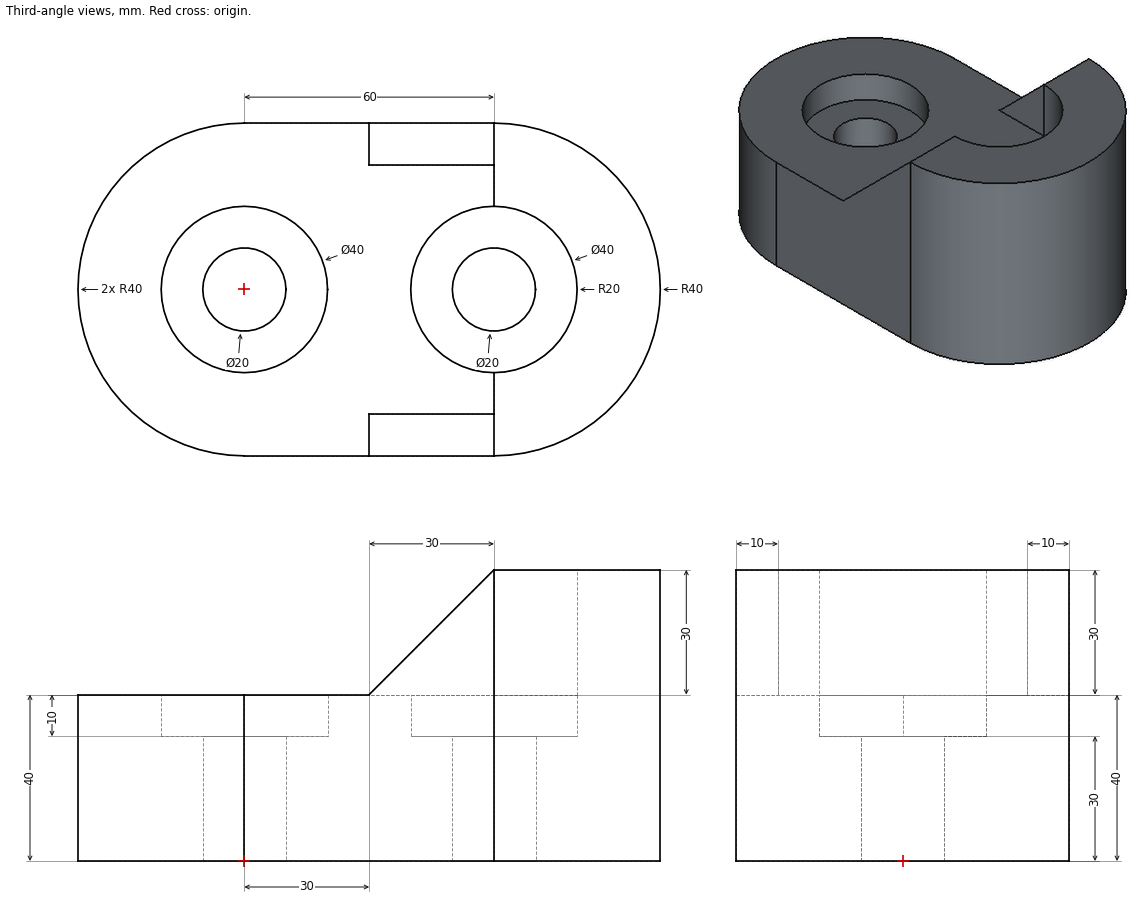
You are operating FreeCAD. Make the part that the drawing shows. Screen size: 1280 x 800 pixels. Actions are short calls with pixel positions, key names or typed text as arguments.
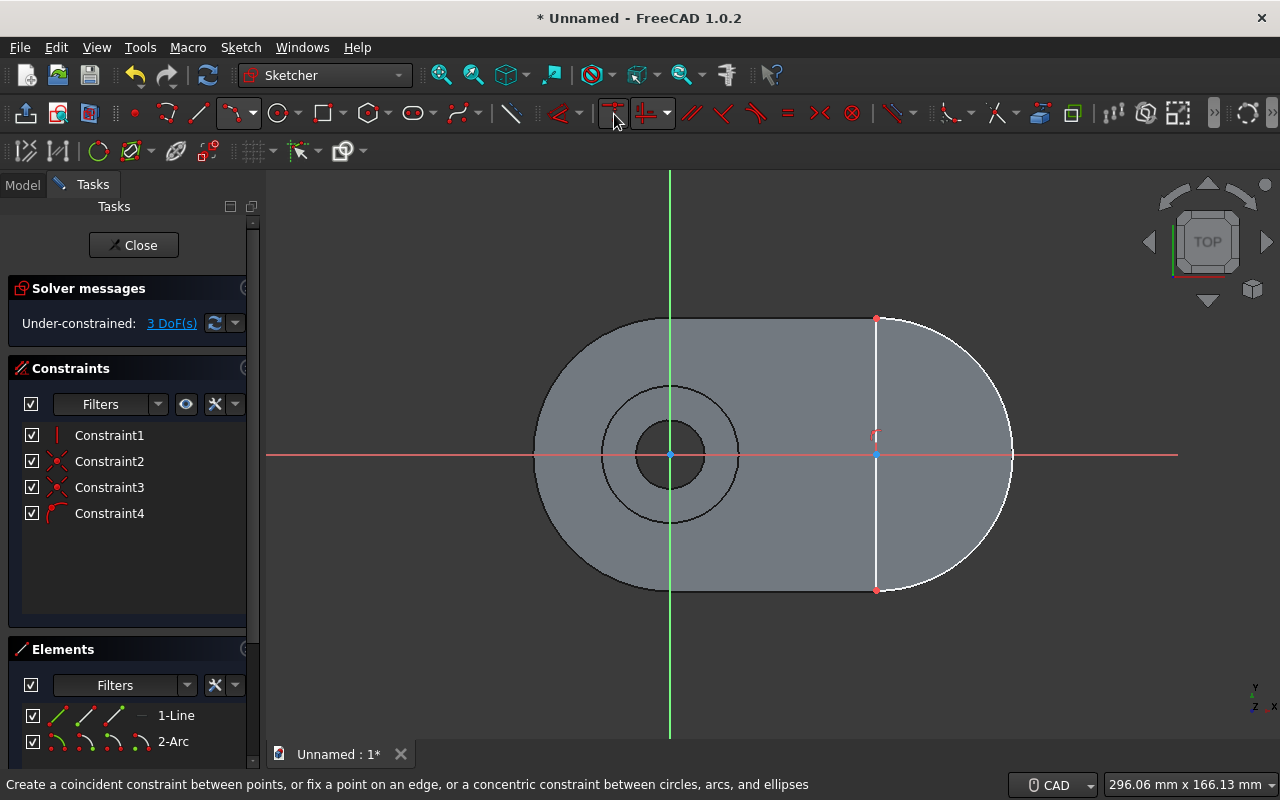
click(558, 114)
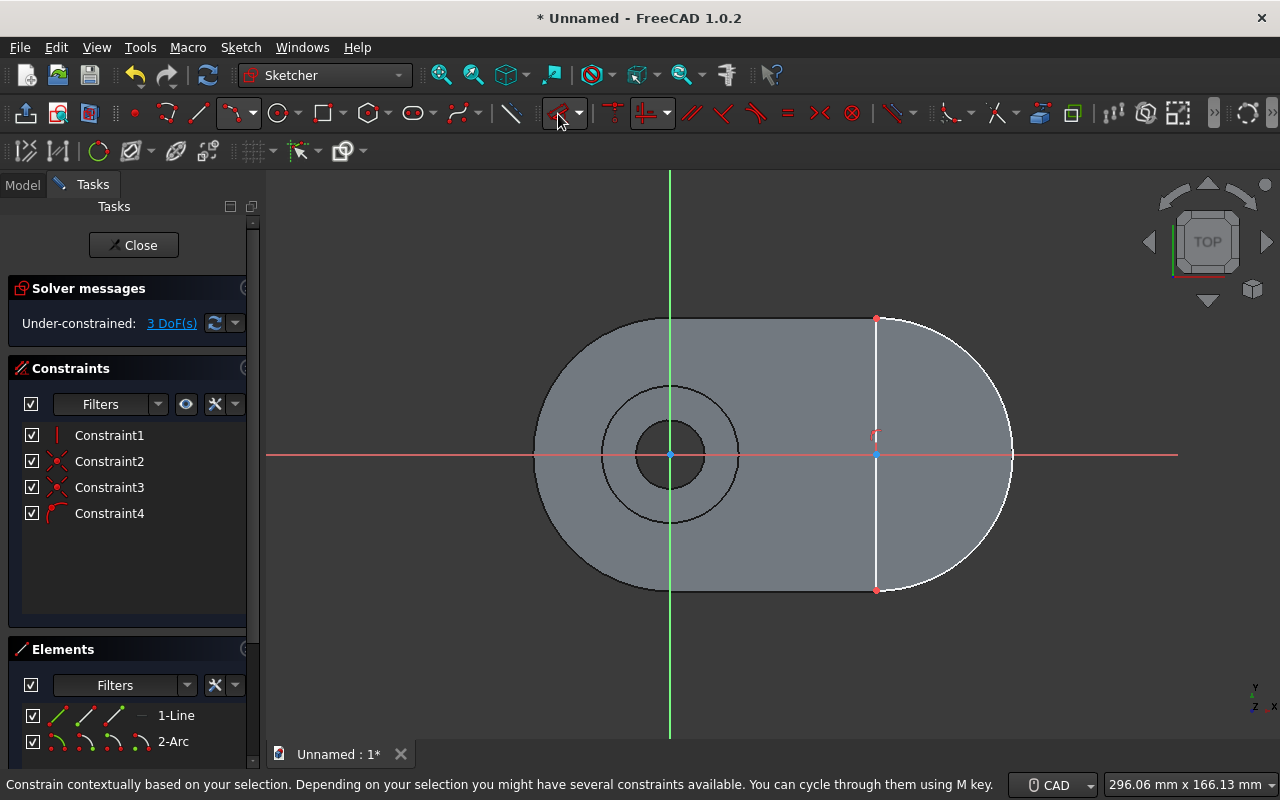
click(987, 535)
click(1013, 554)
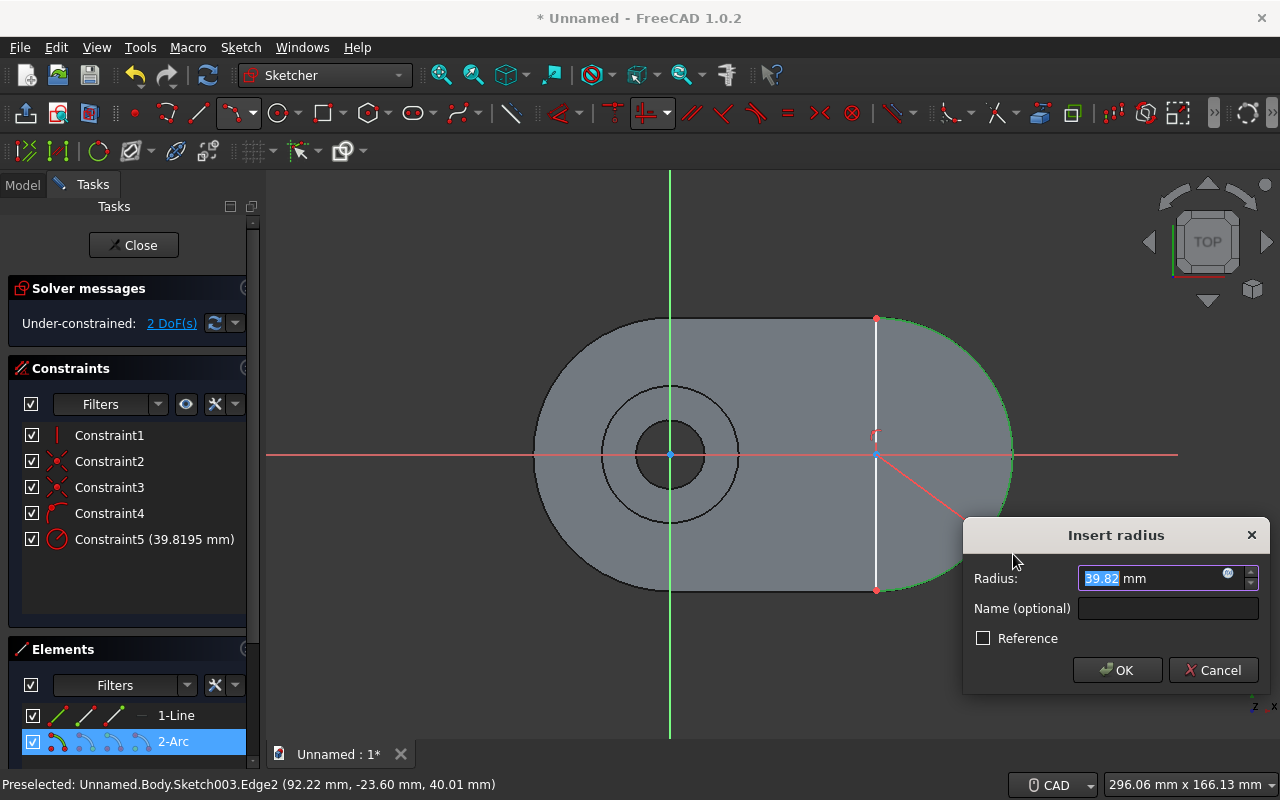
text(40)
key(Return)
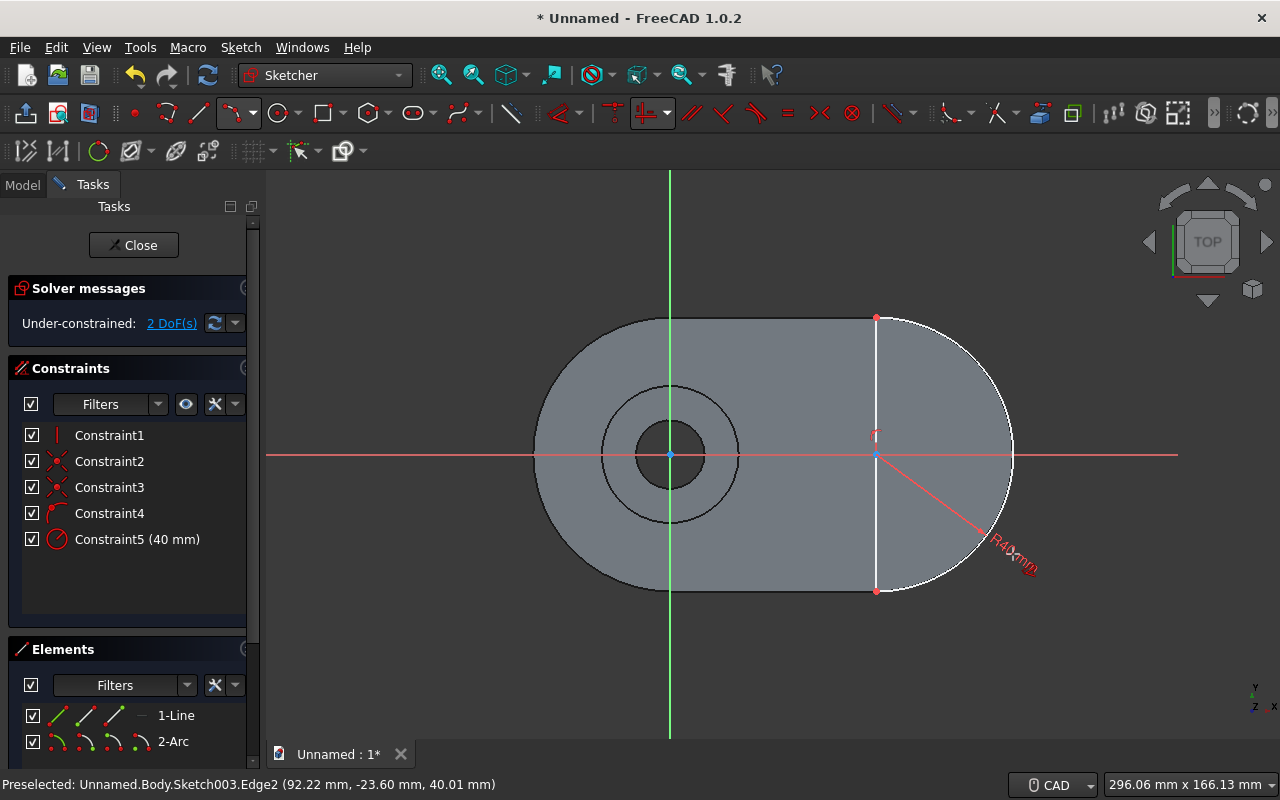
click(876, 318)
click(773, 284)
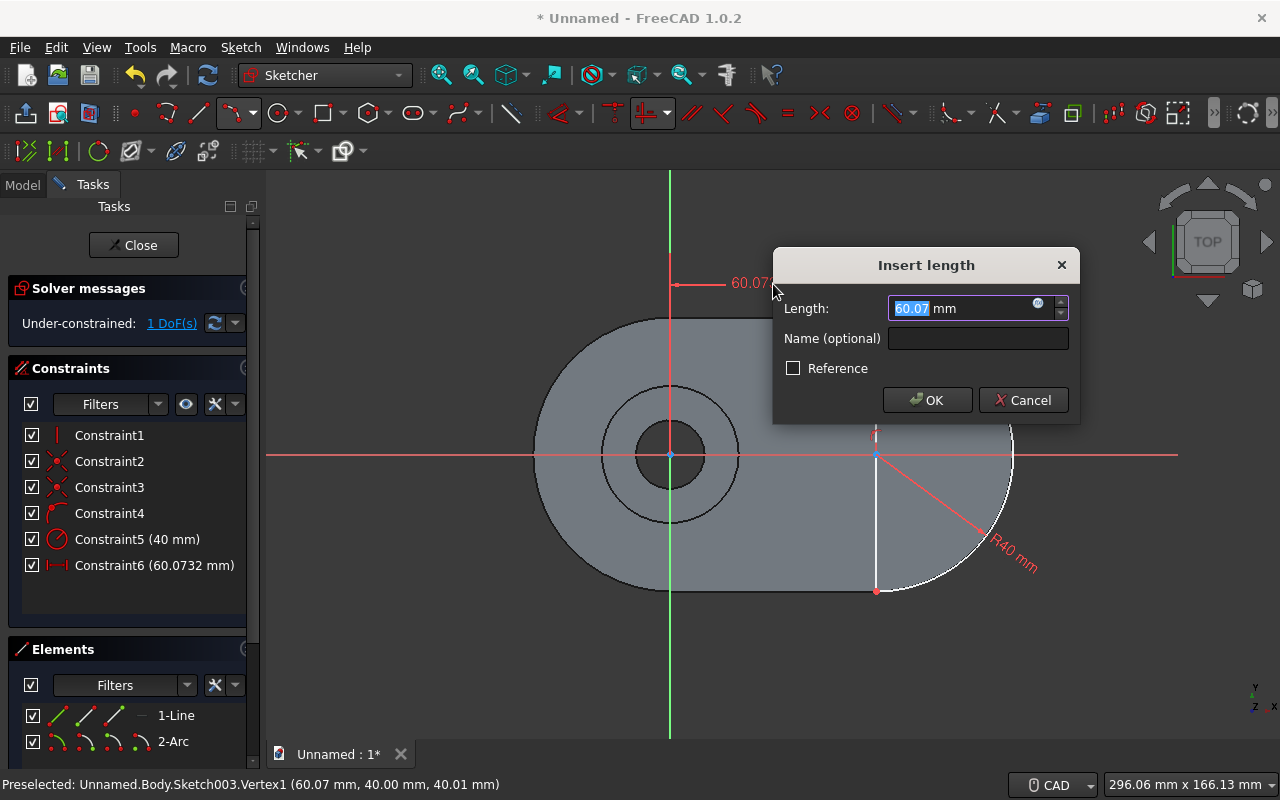
text(60)
key(Return)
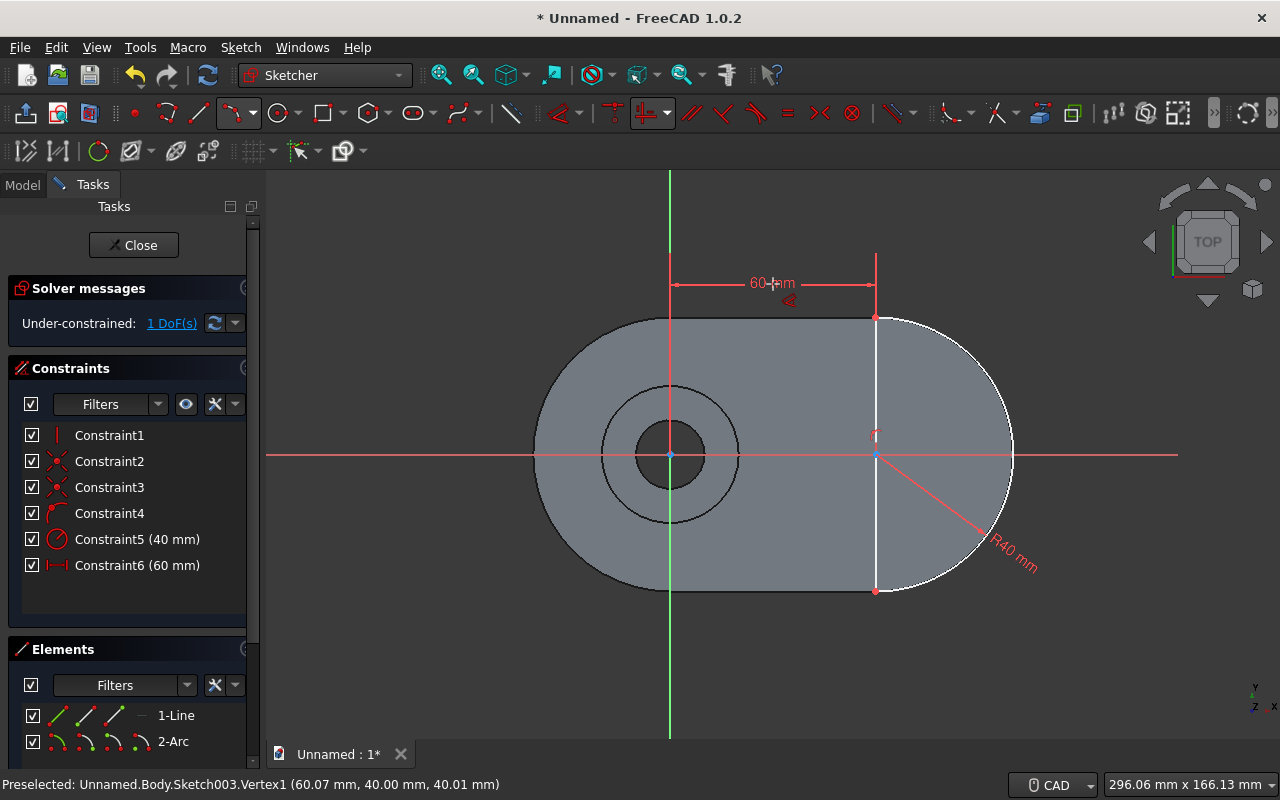
click(876, 455)
click(773, 489)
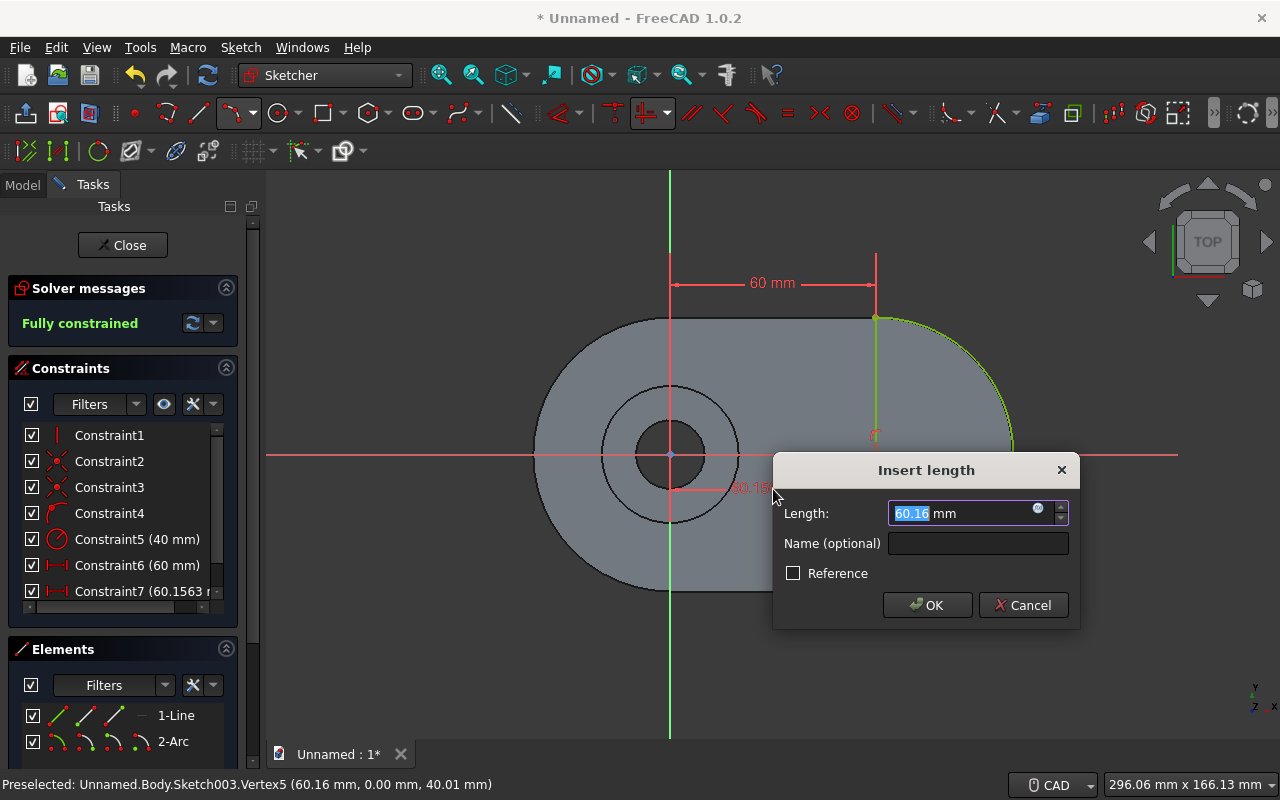
text(60)
key(Return)
key(Escape)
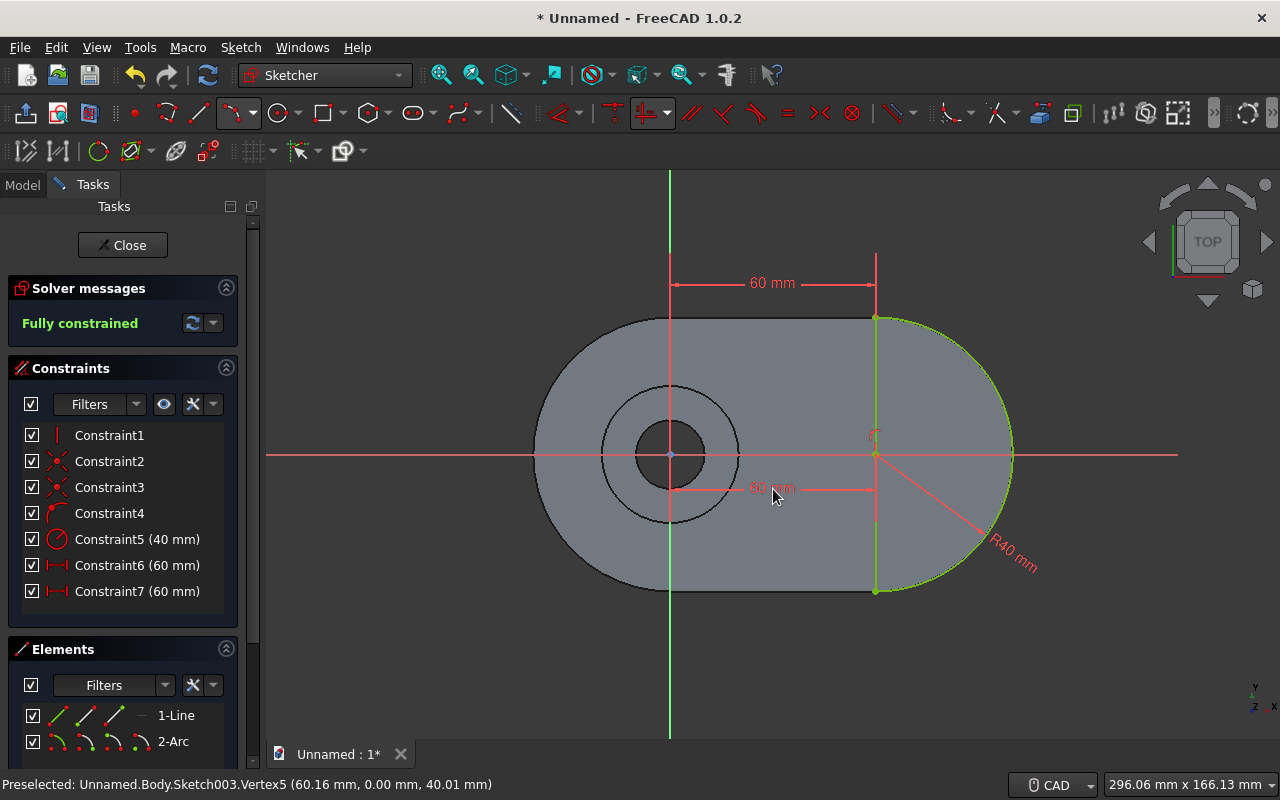
click(123, 245)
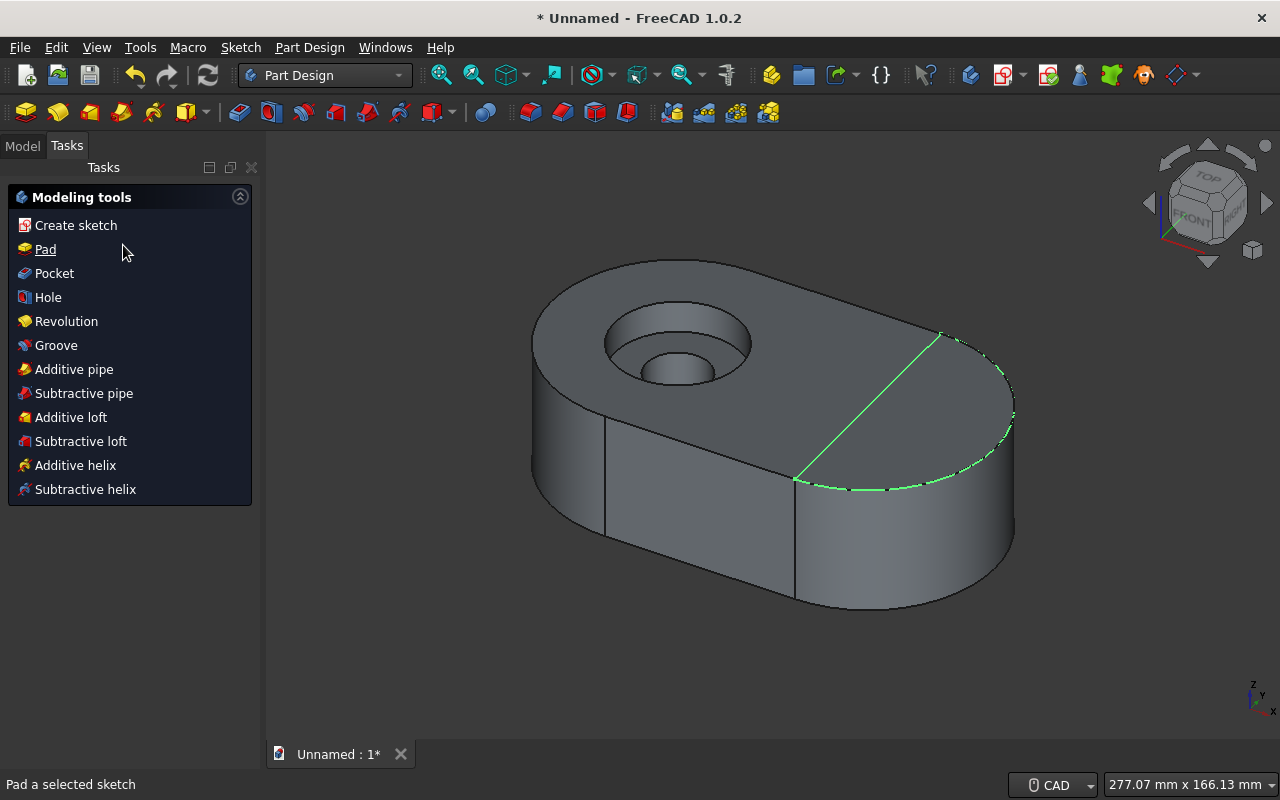
click(26, 112)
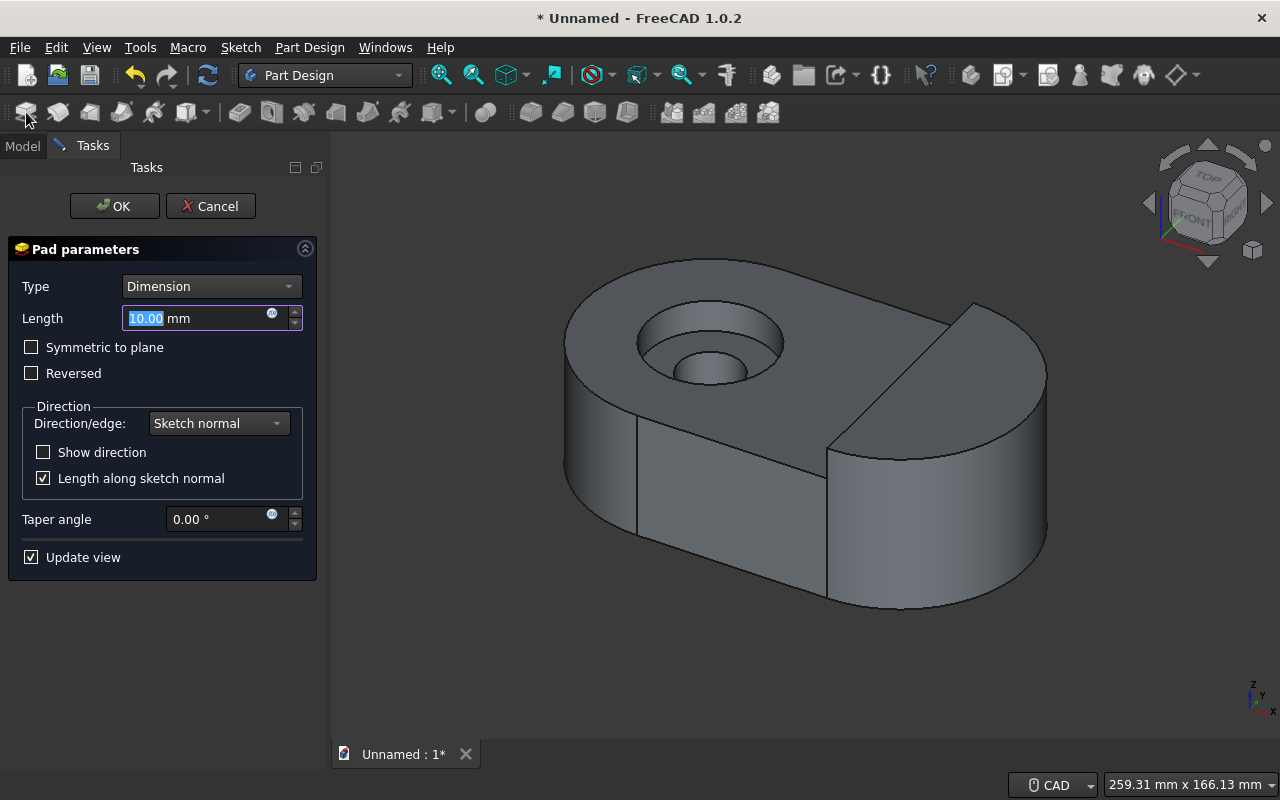
text(30)
key(Tab)